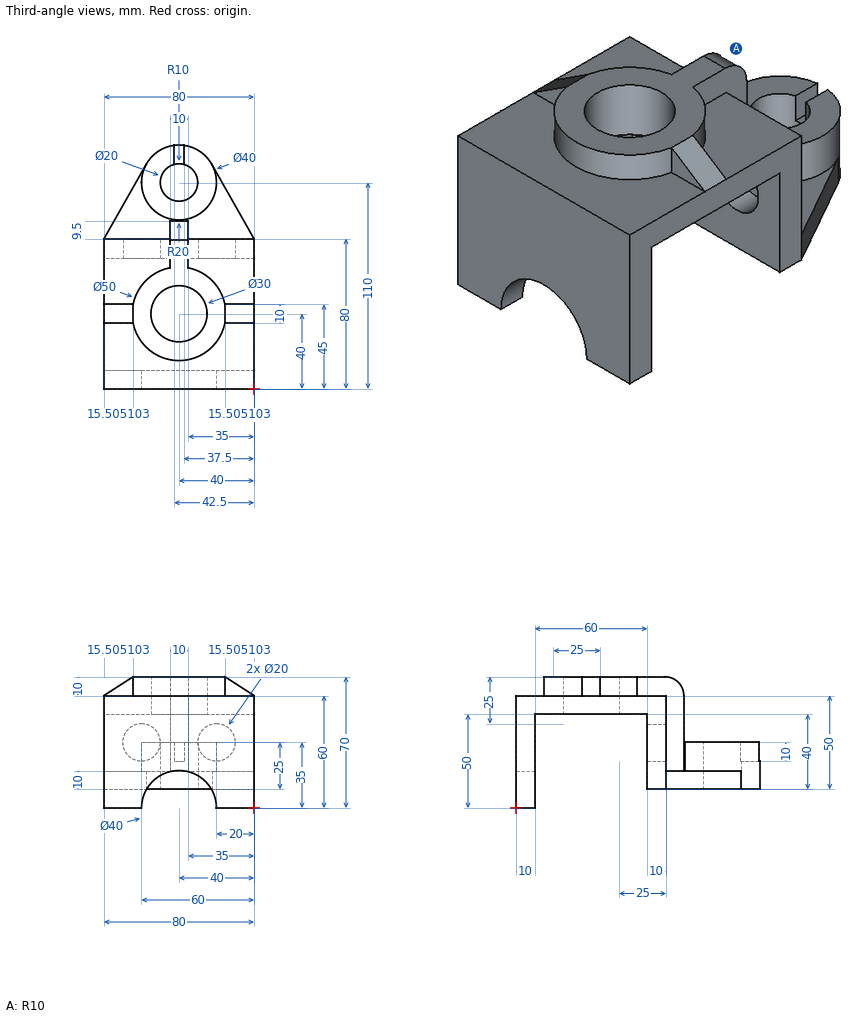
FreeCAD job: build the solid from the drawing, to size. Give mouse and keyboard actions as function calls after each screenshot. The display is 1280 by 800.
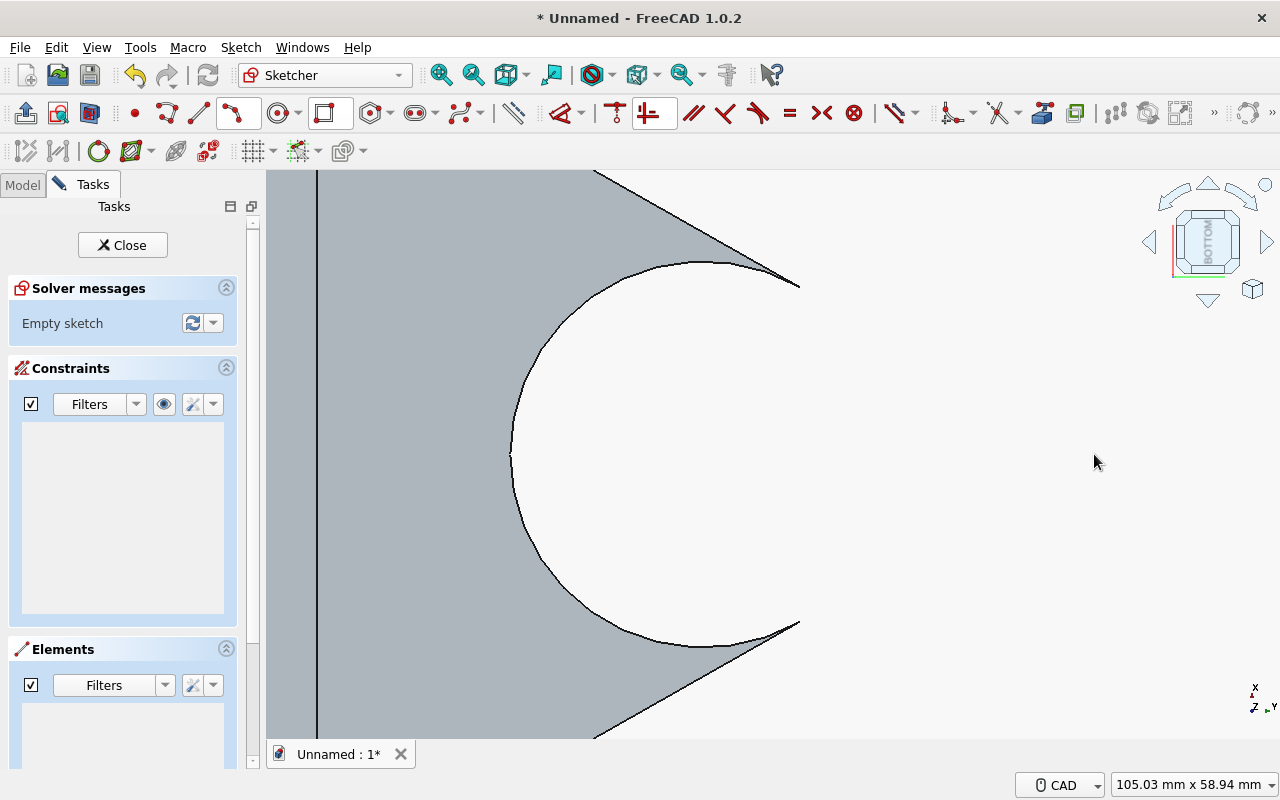
click(278, 114)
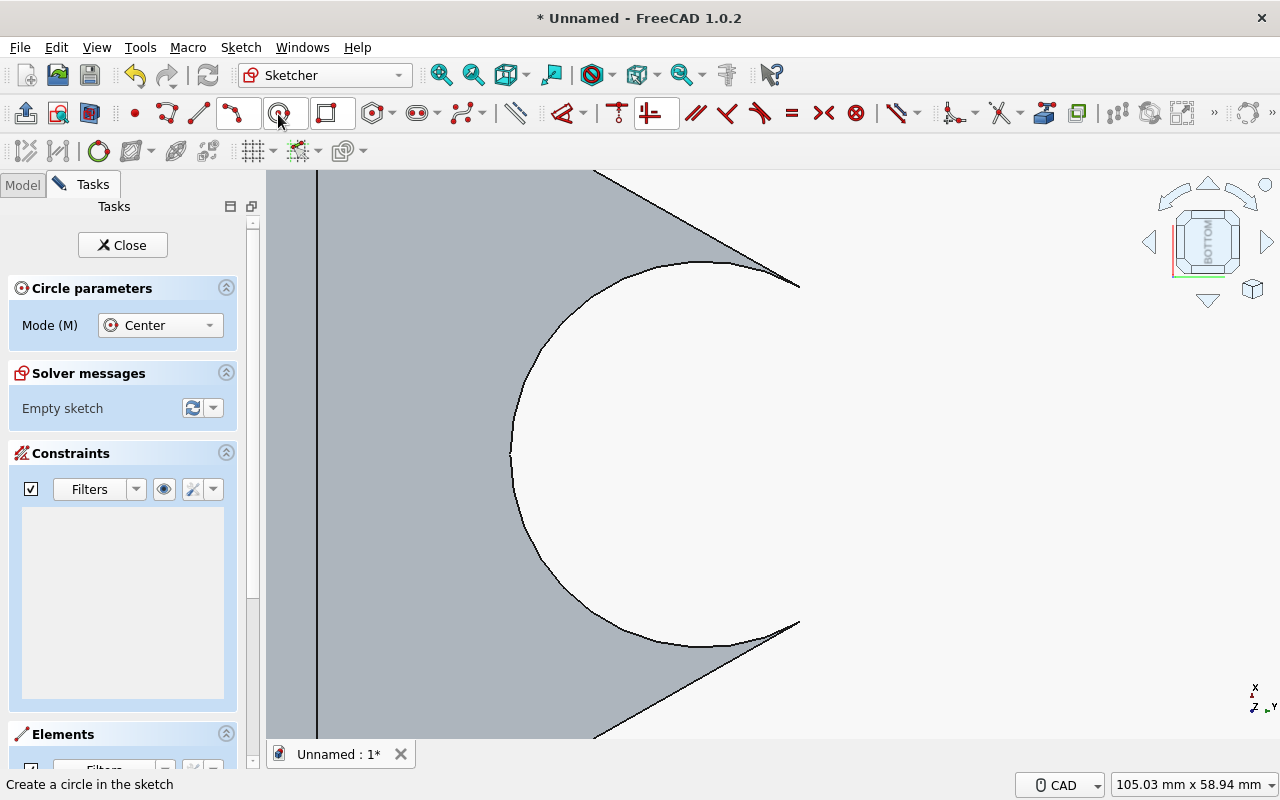
click(703, 454)
move(840, 318)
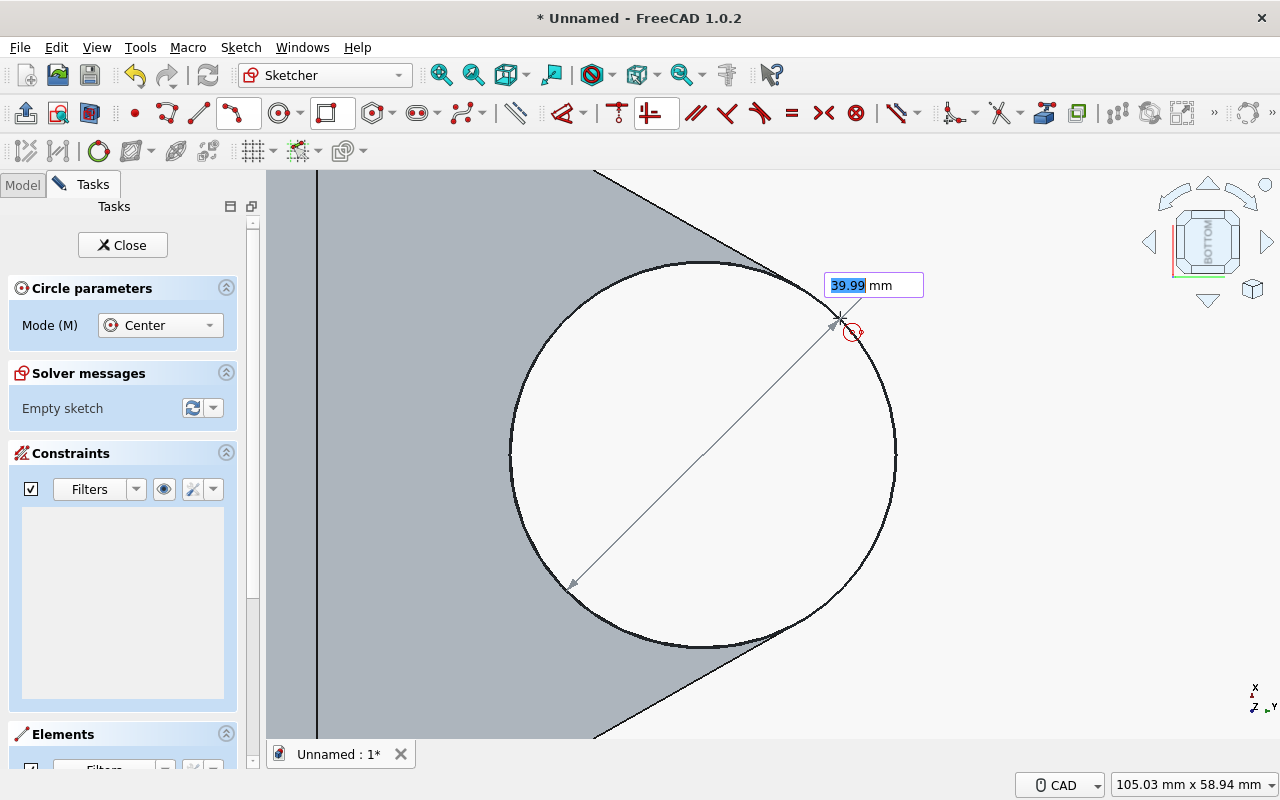
text(40)
key(Return)
key(Escape)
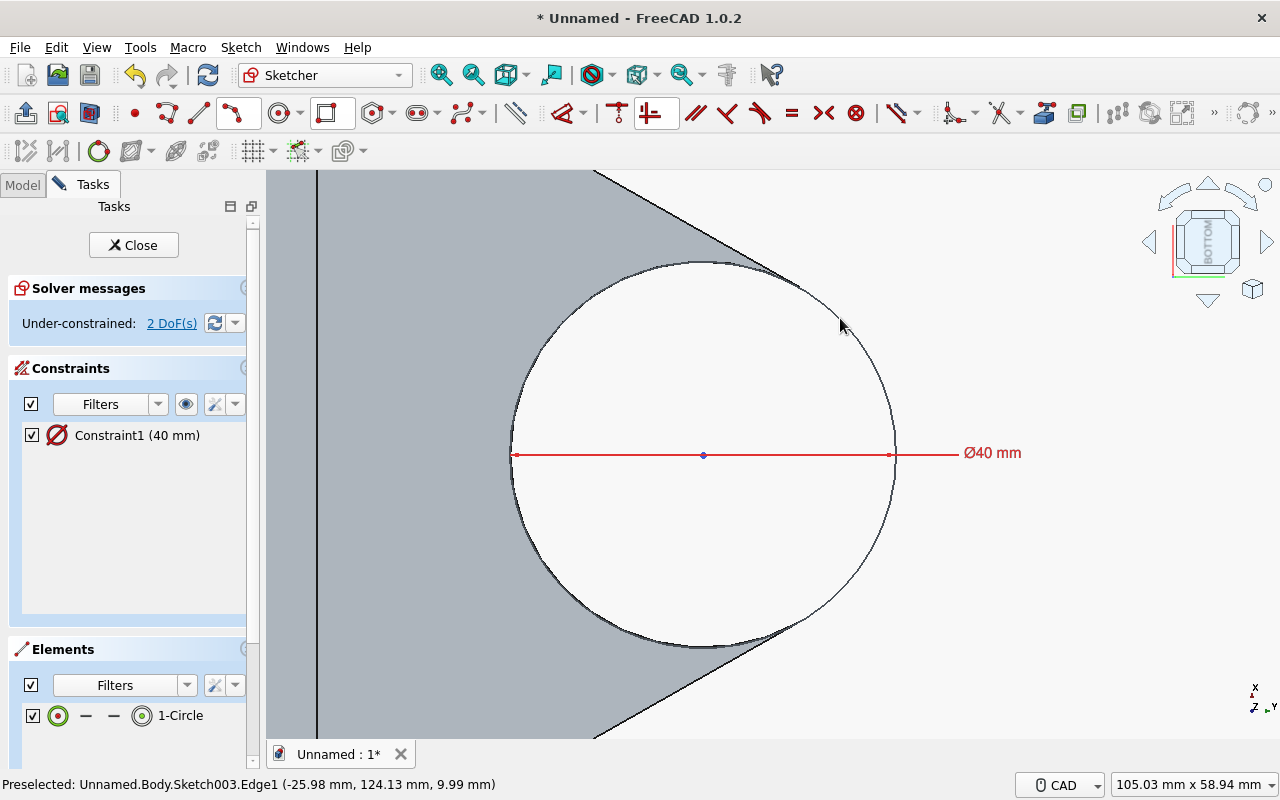
click(562, 114)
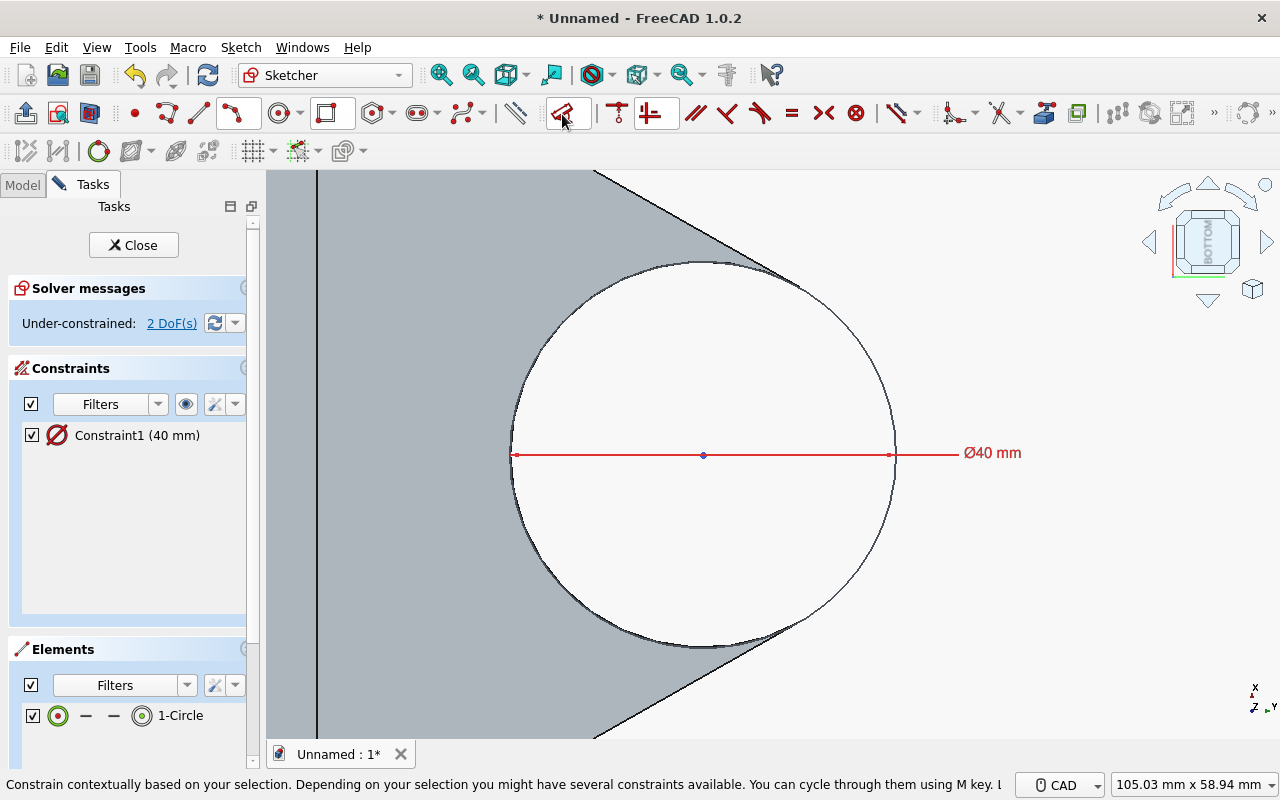
click(703, 455)
click(737, 327)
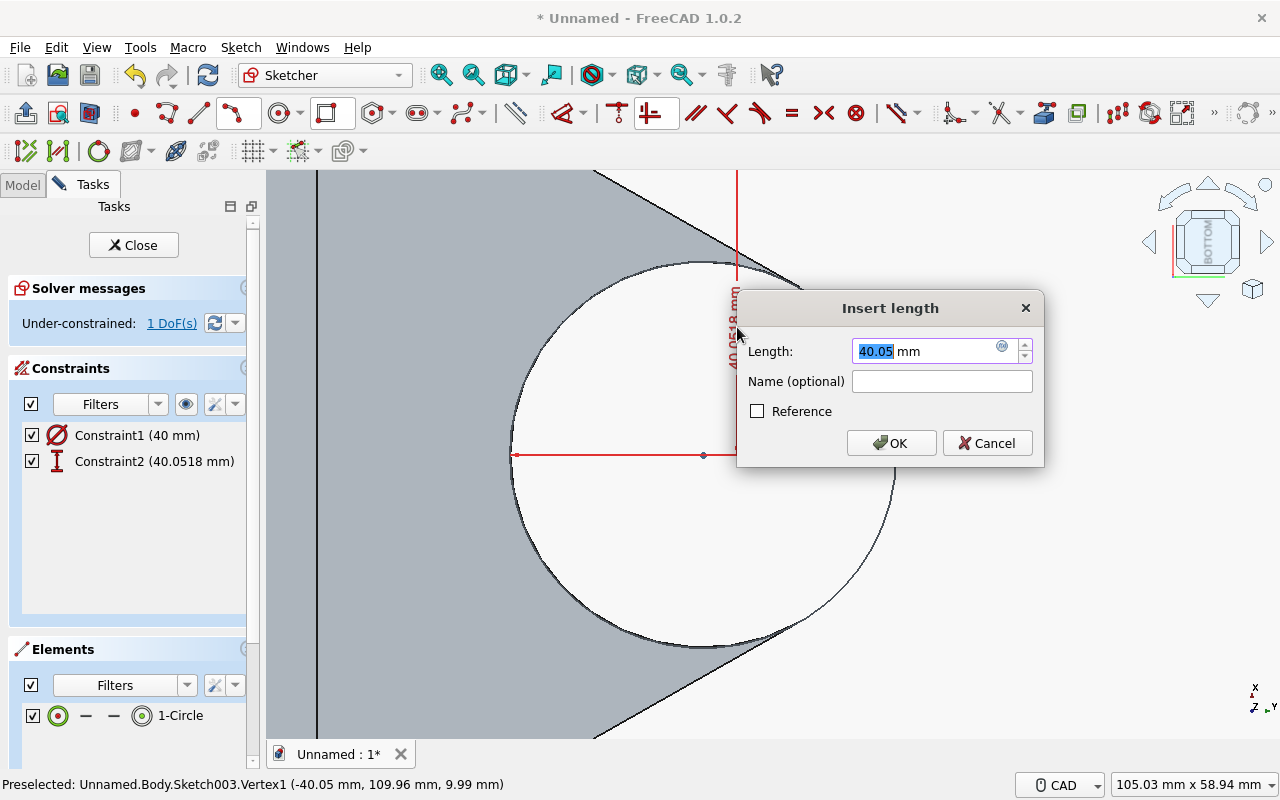
text(40)
key(Return)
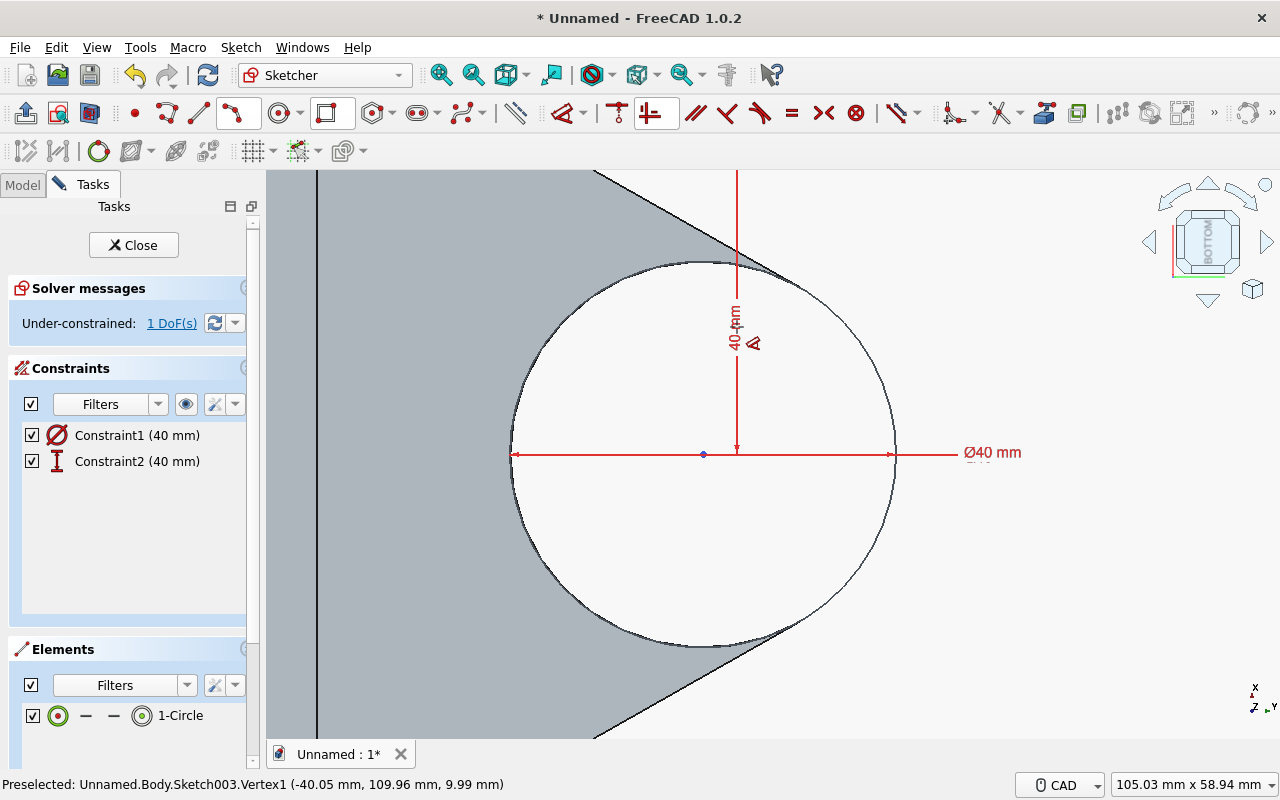
click(703, 454)
click(498, 488)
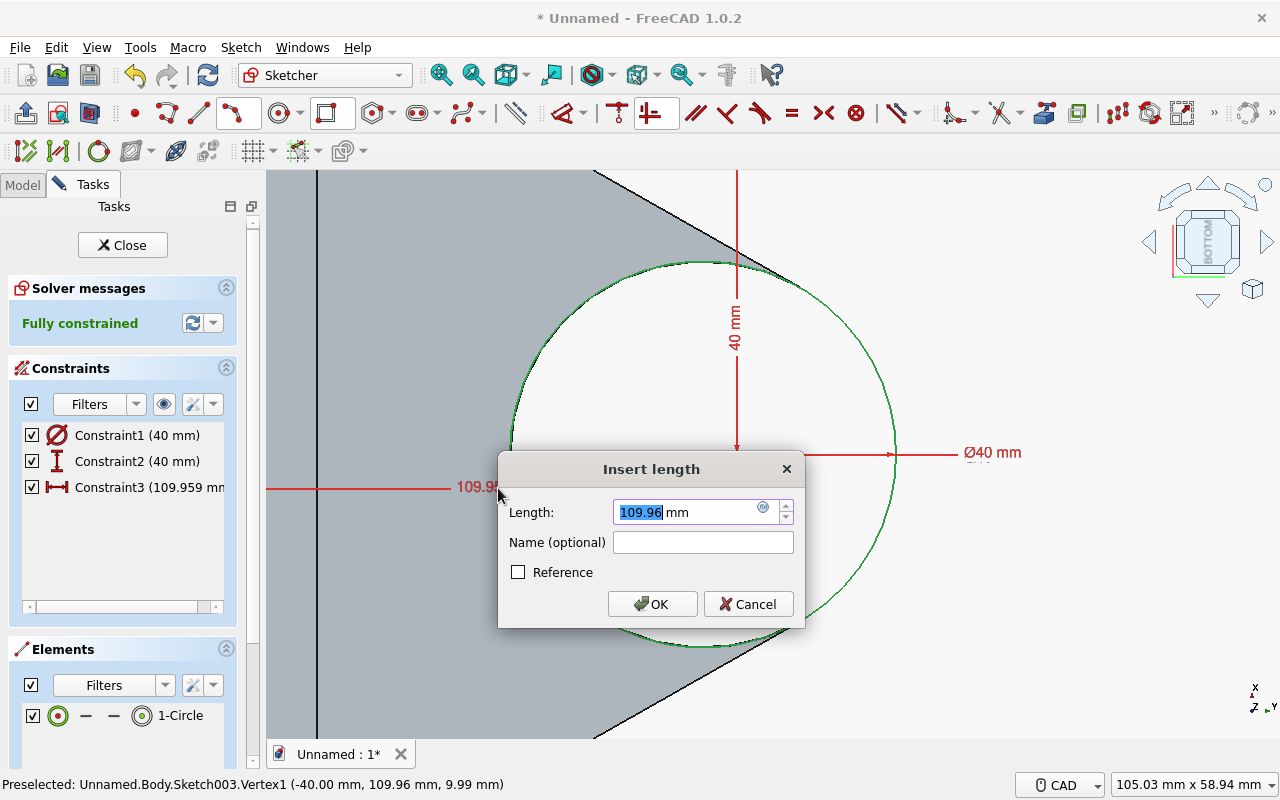
text(110)
key(Return)
key(Escape)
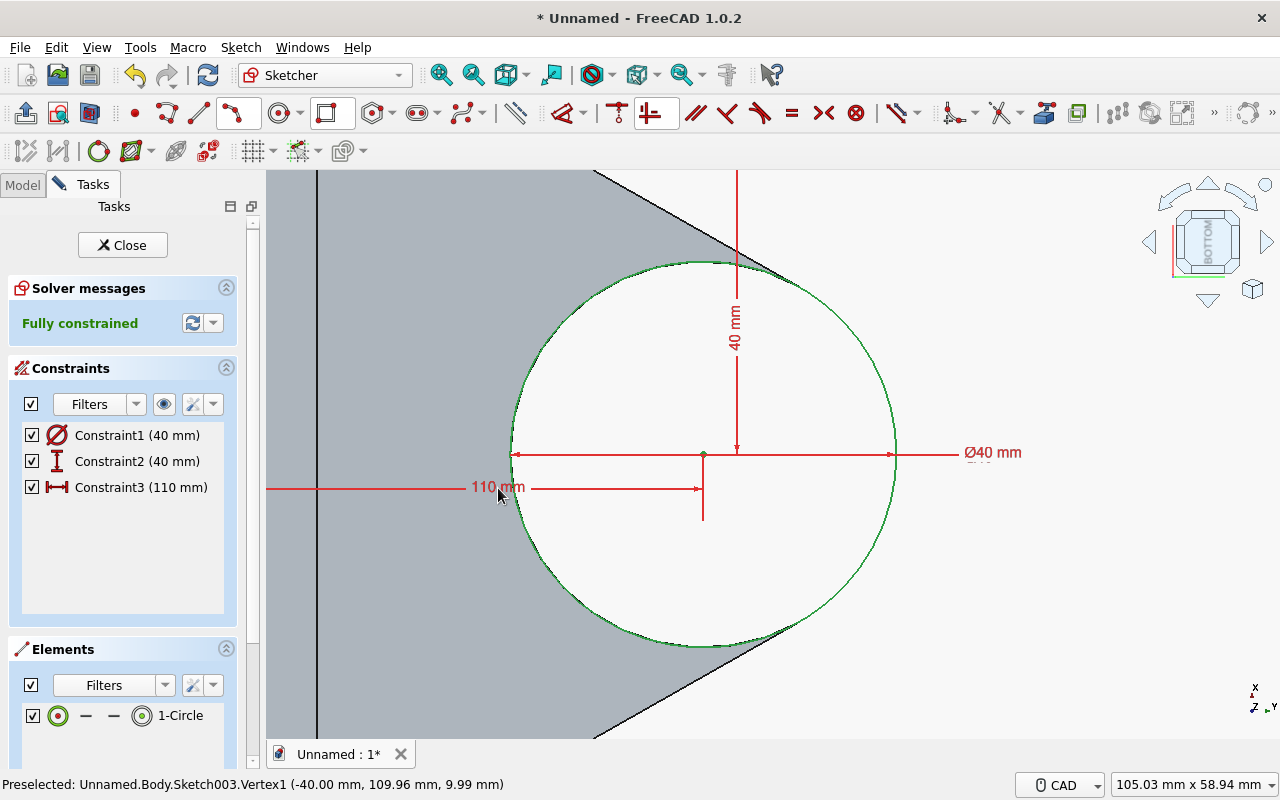
click(123, 245)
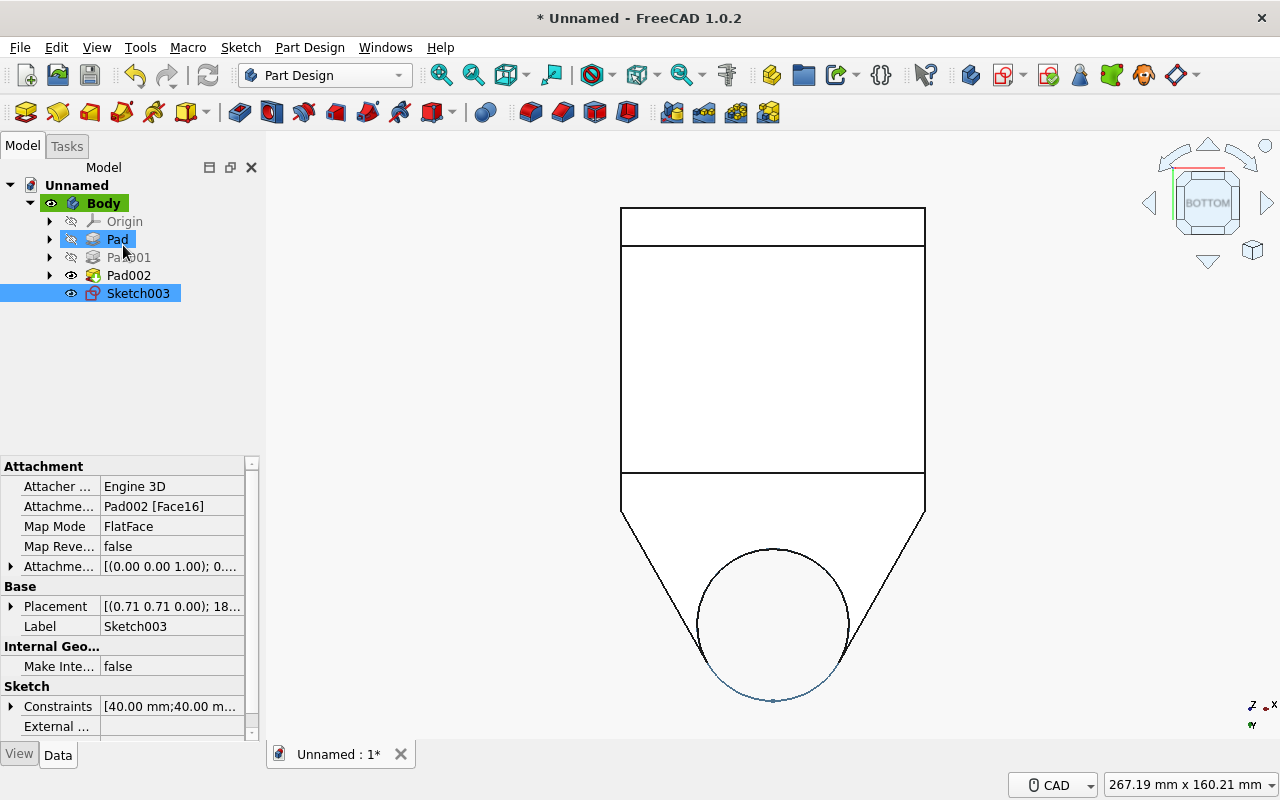
click(26, 112)